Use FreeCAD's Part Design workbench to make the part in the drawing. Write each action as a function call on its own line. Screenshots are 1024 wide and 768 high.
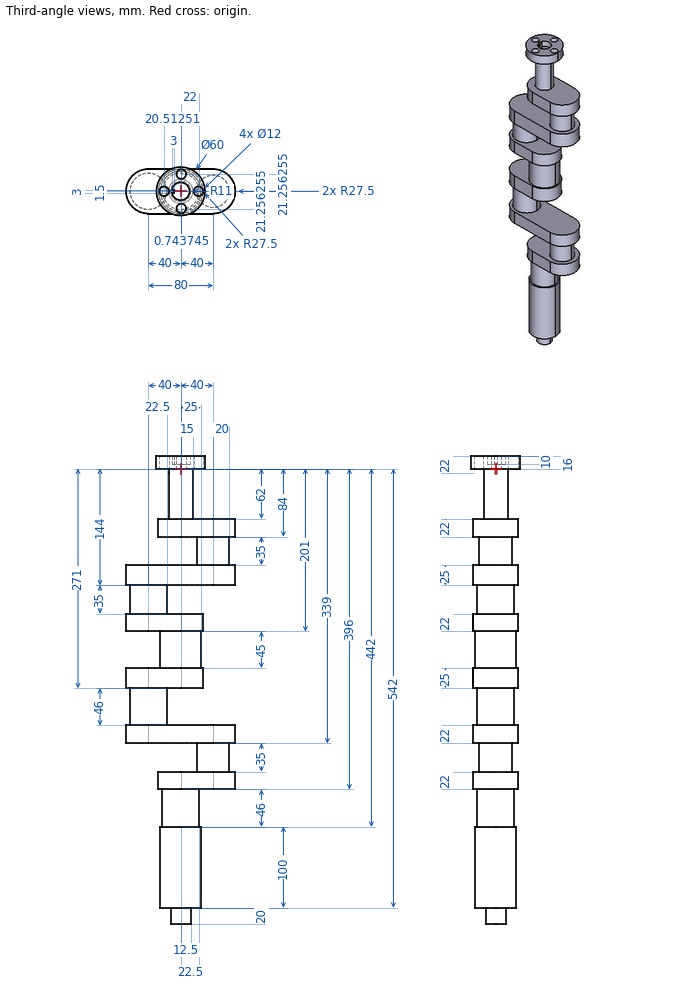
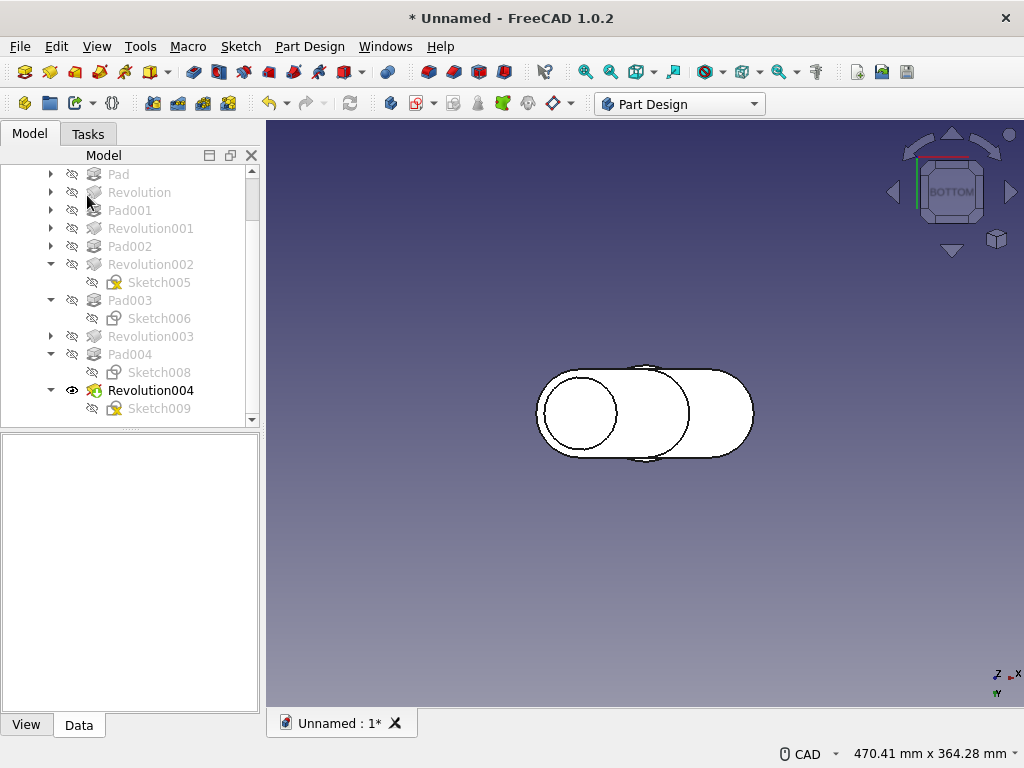
click(581, 412)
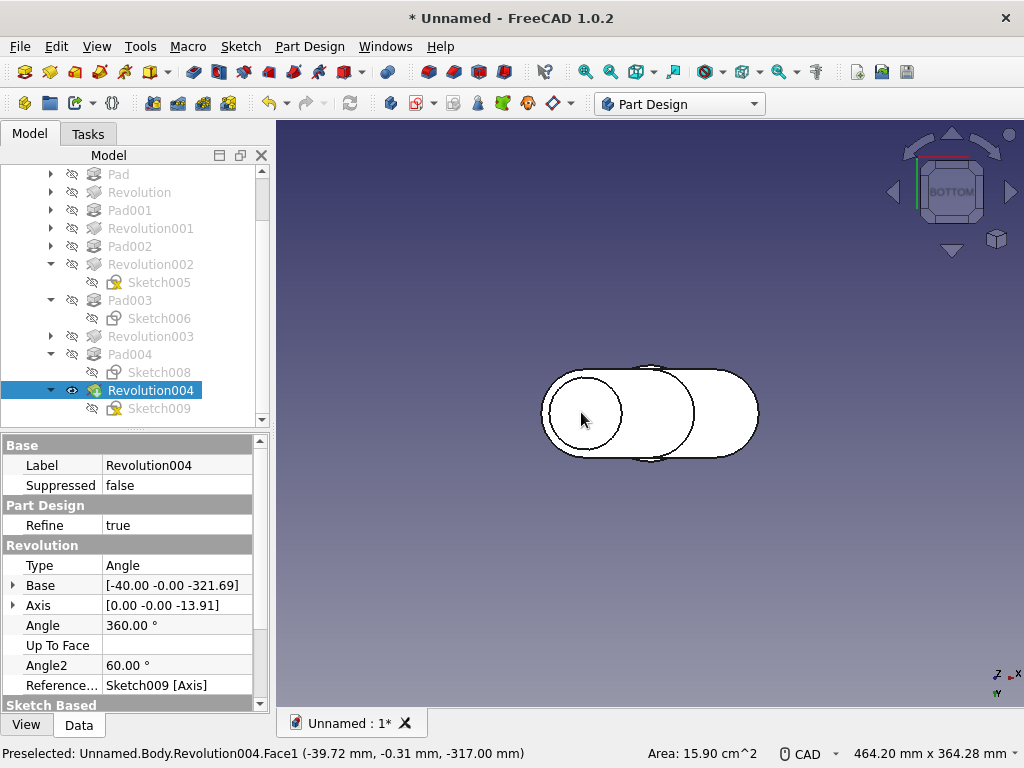
click(416, 104)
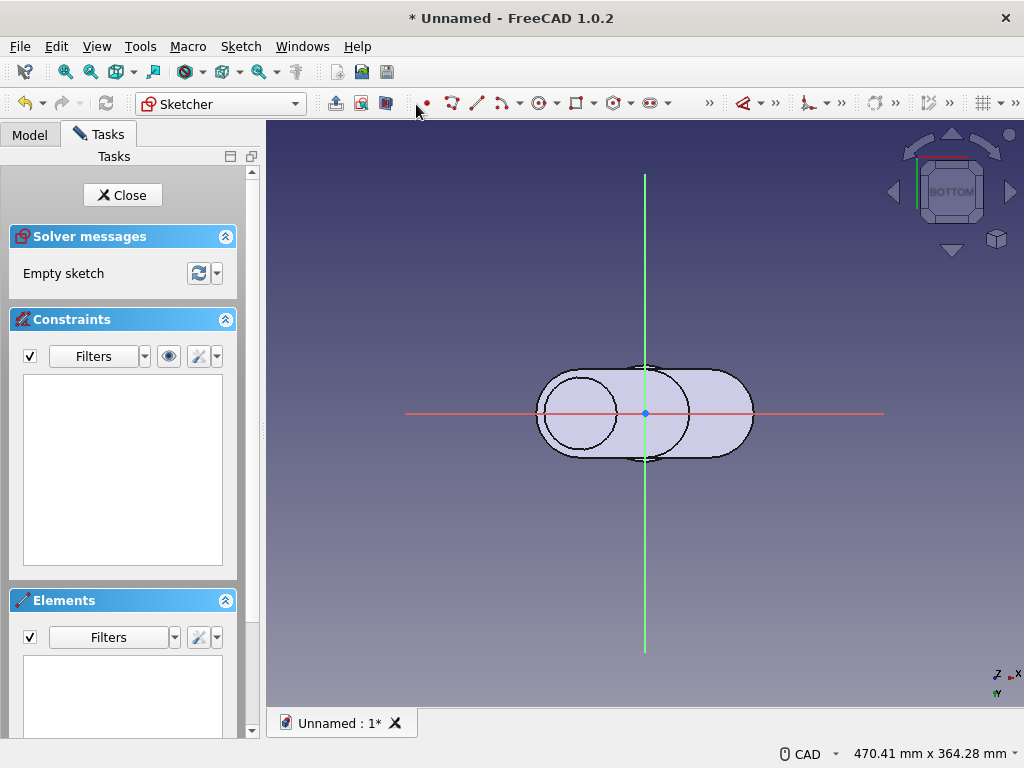
scroll(728, 413, up, 3)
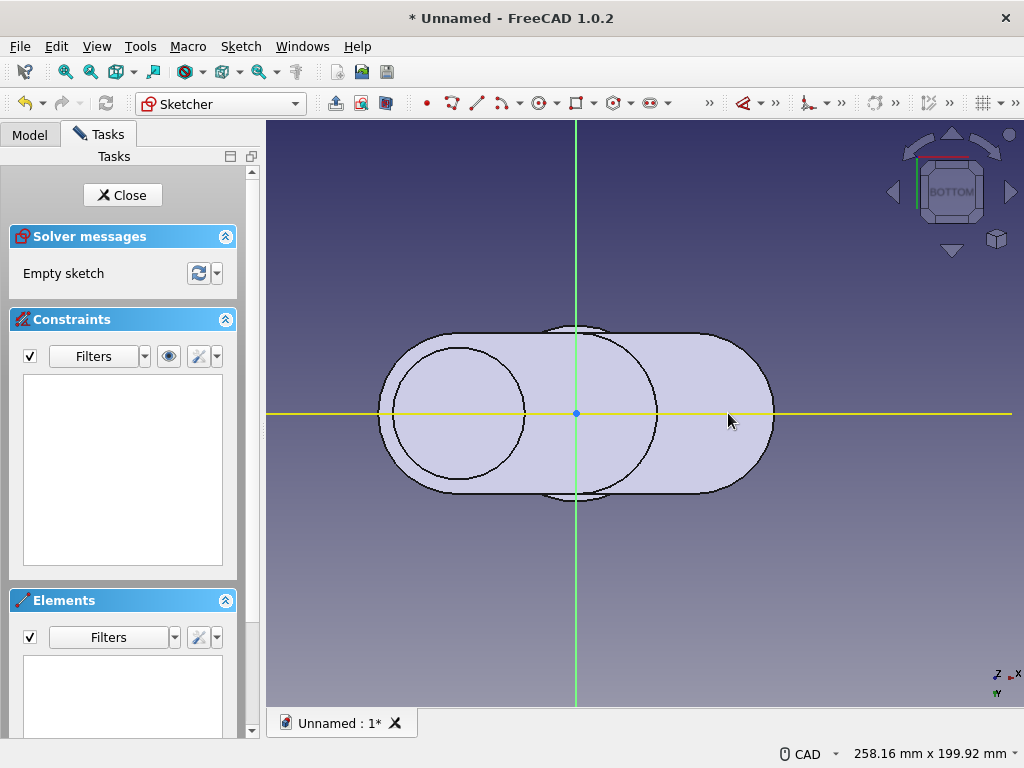
key(g)
key(s)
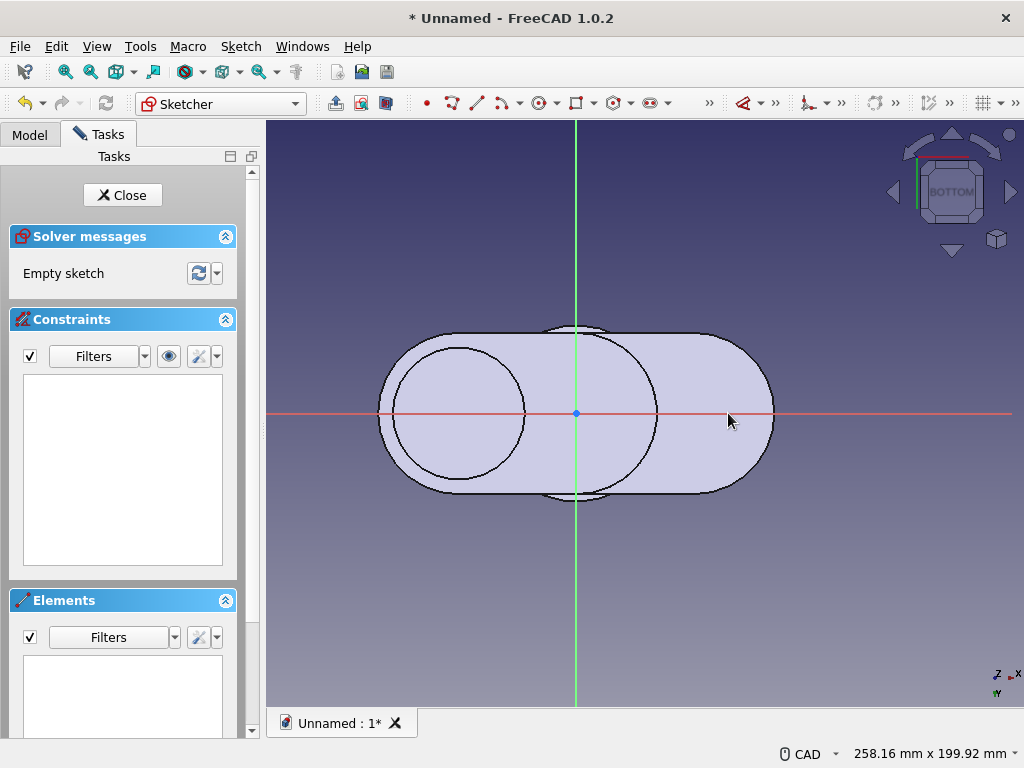
click(459, 413)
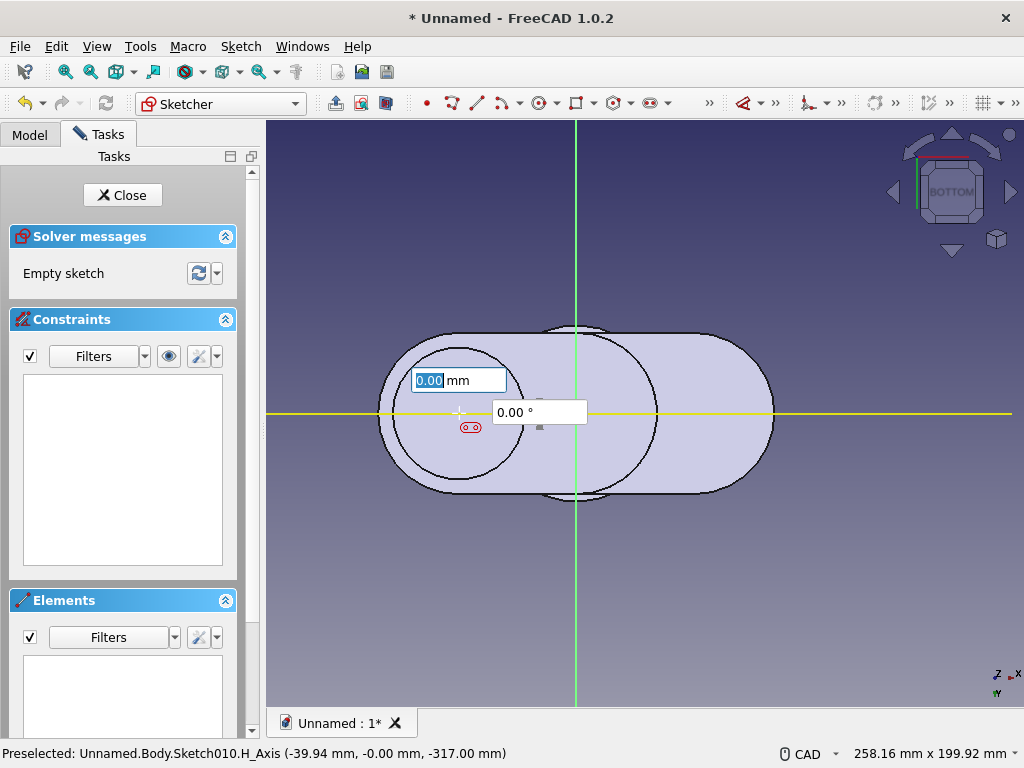
click(694, 404)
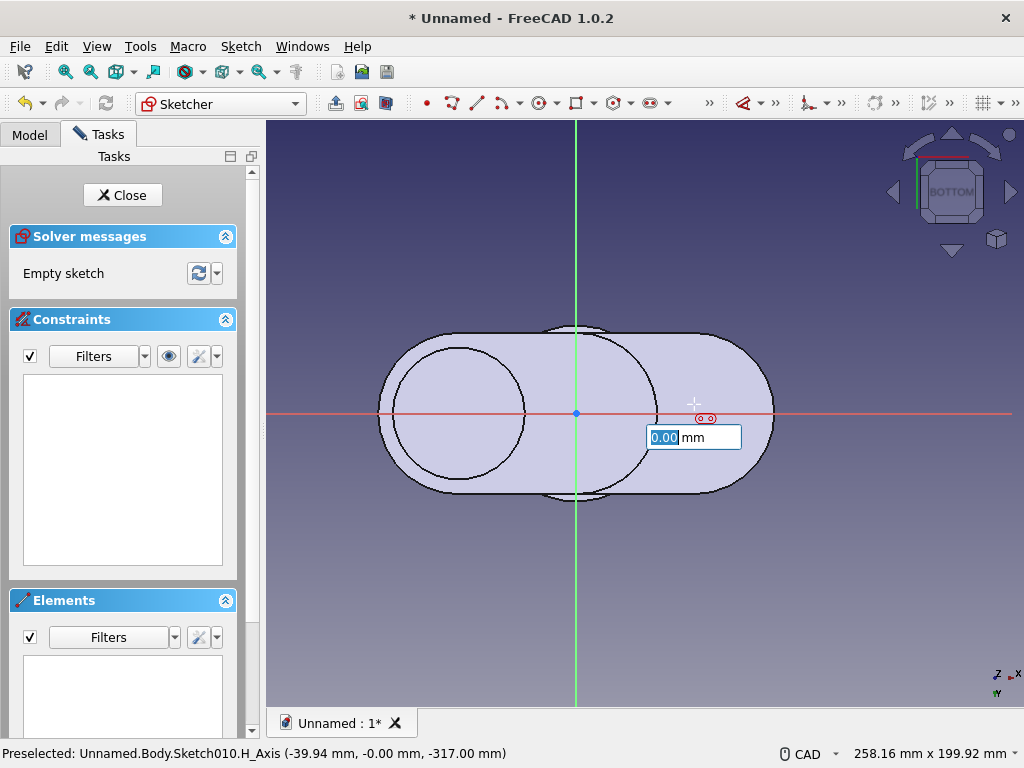
click(541, 494)
key(Escape)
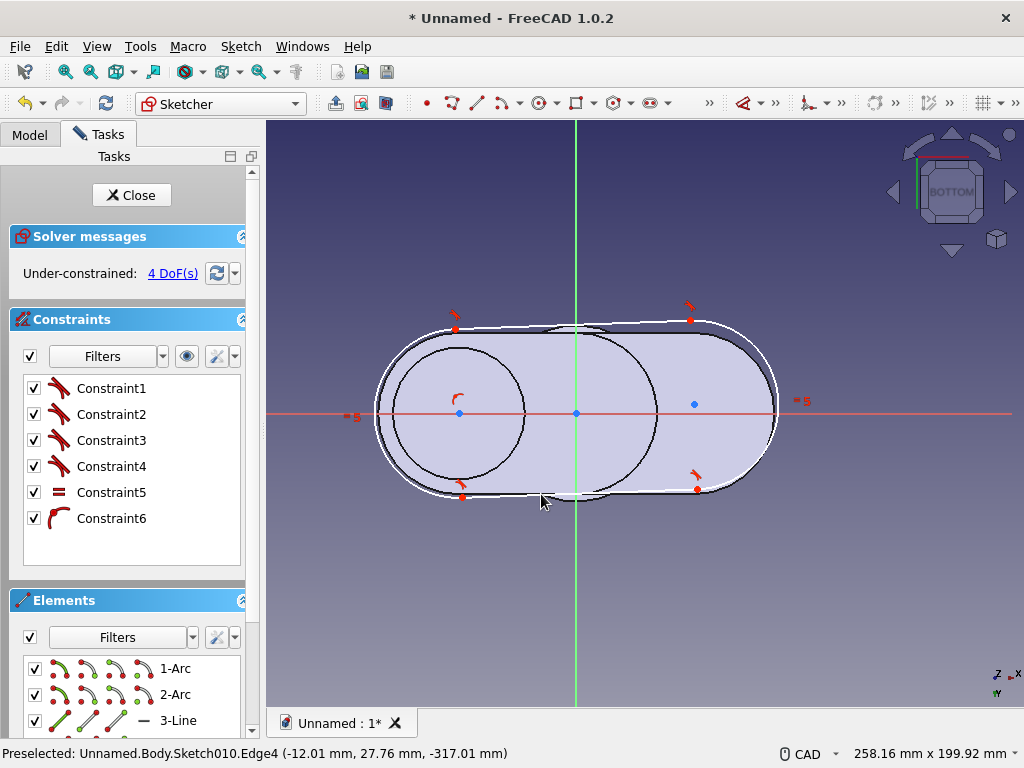
click(526, 327)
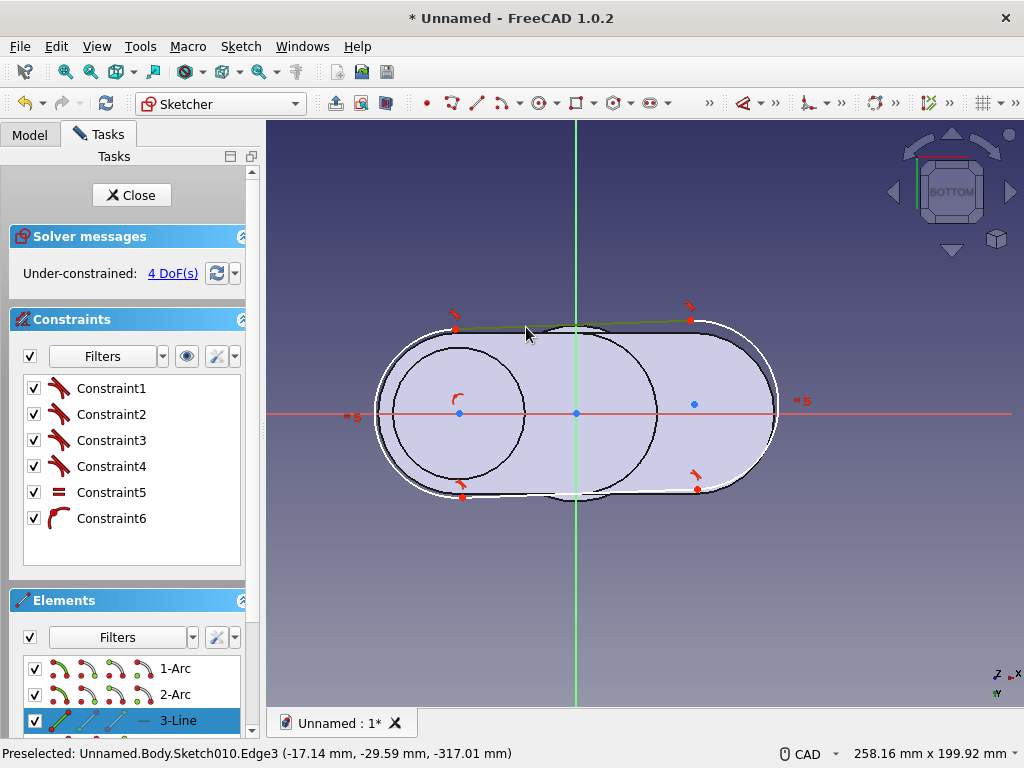
key(h)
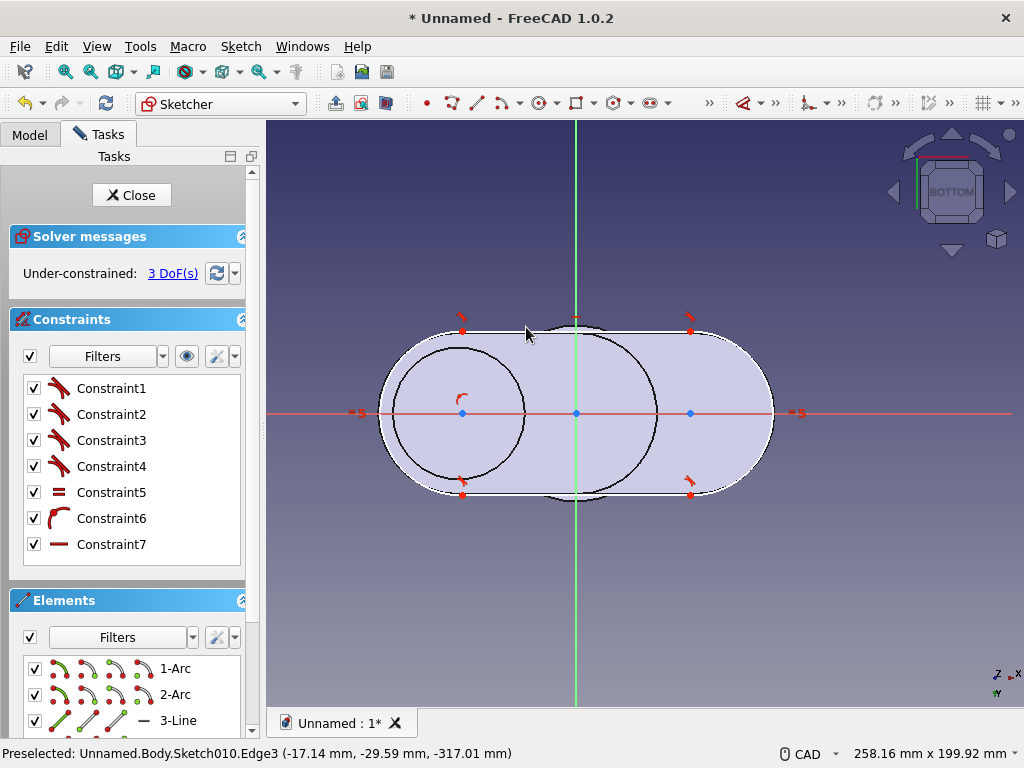
key(d)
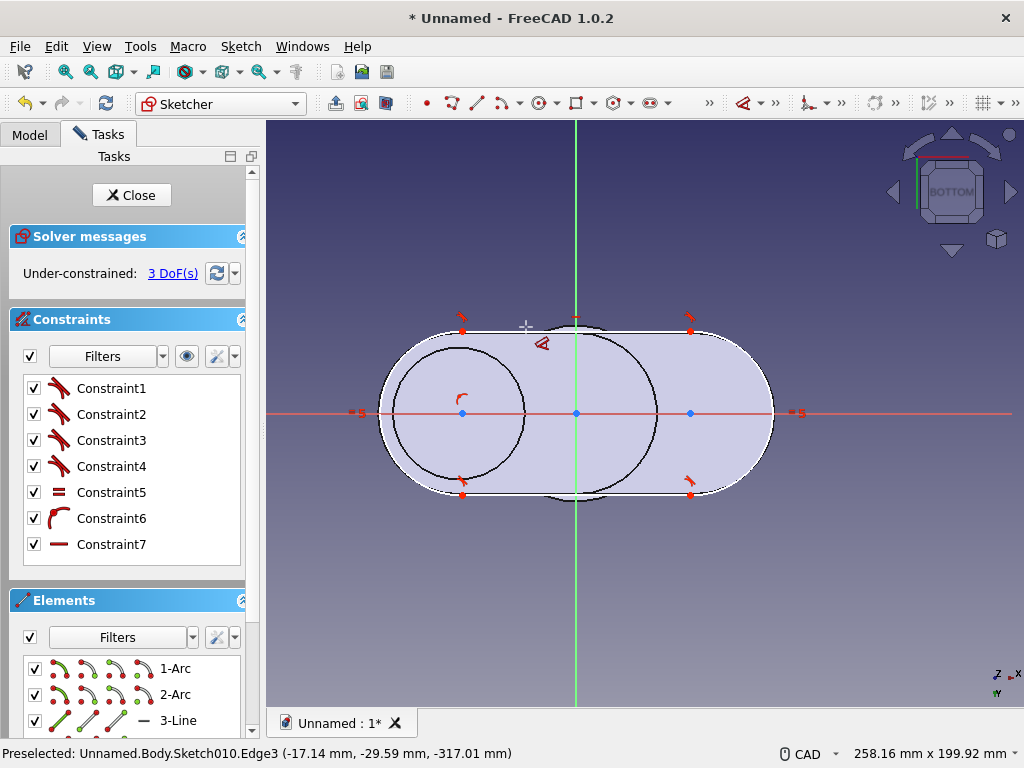
click(396, 365)
click(370, 346)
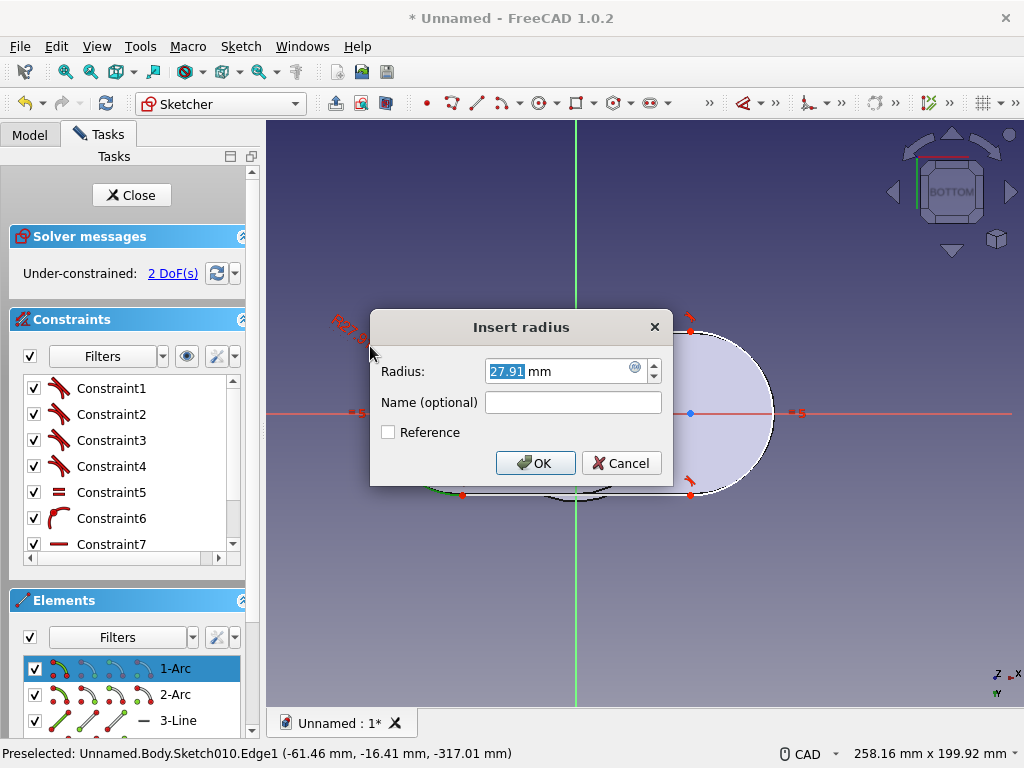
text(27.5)
key(Return)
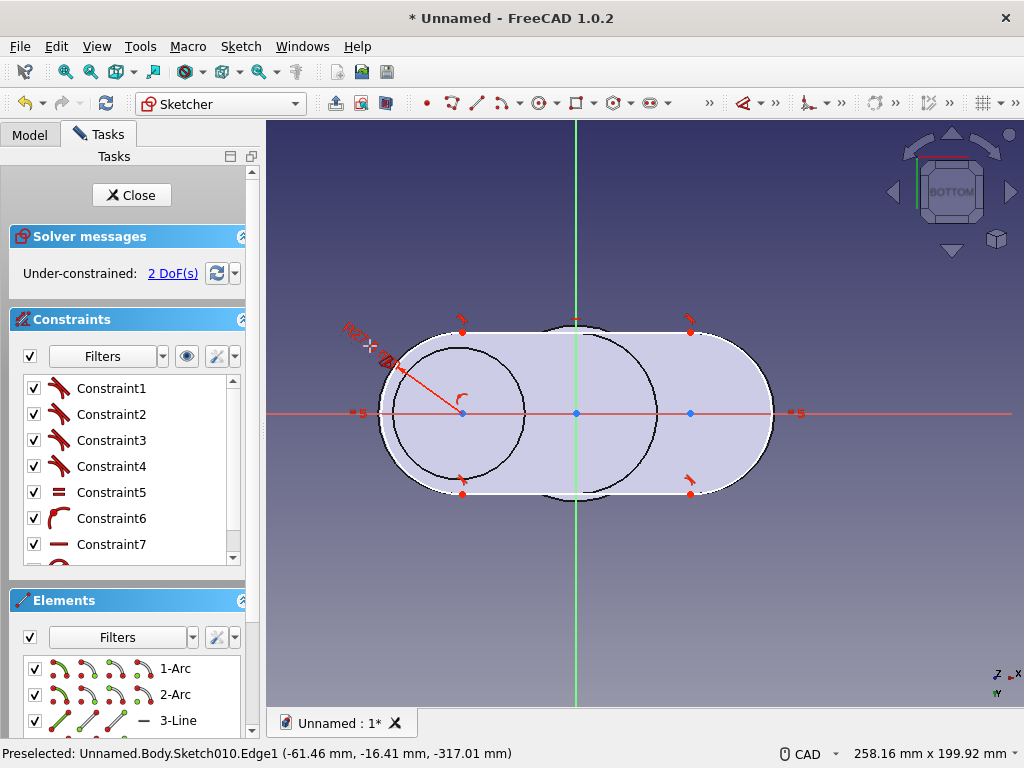
click(531, 333)
click(524, 299)